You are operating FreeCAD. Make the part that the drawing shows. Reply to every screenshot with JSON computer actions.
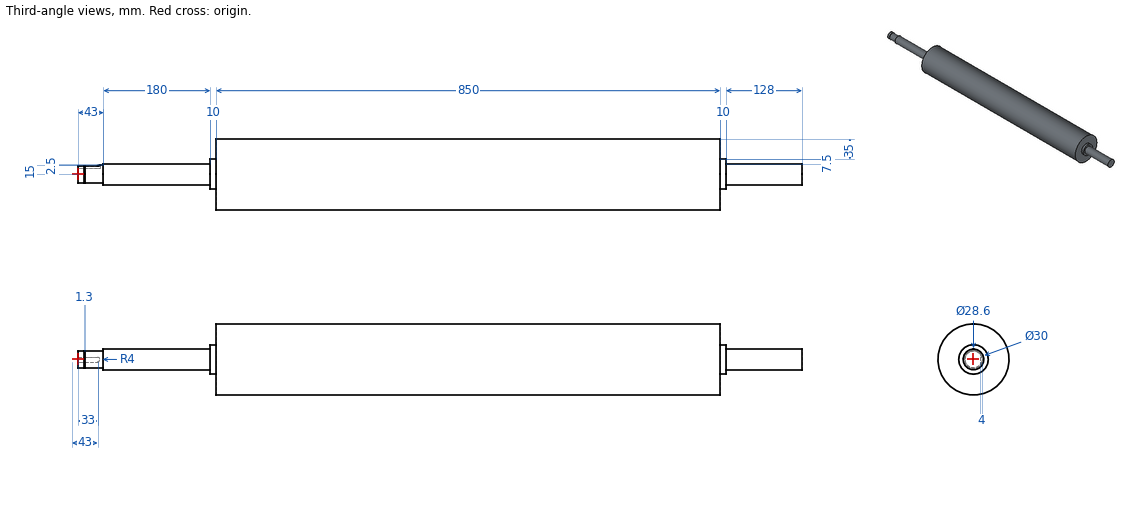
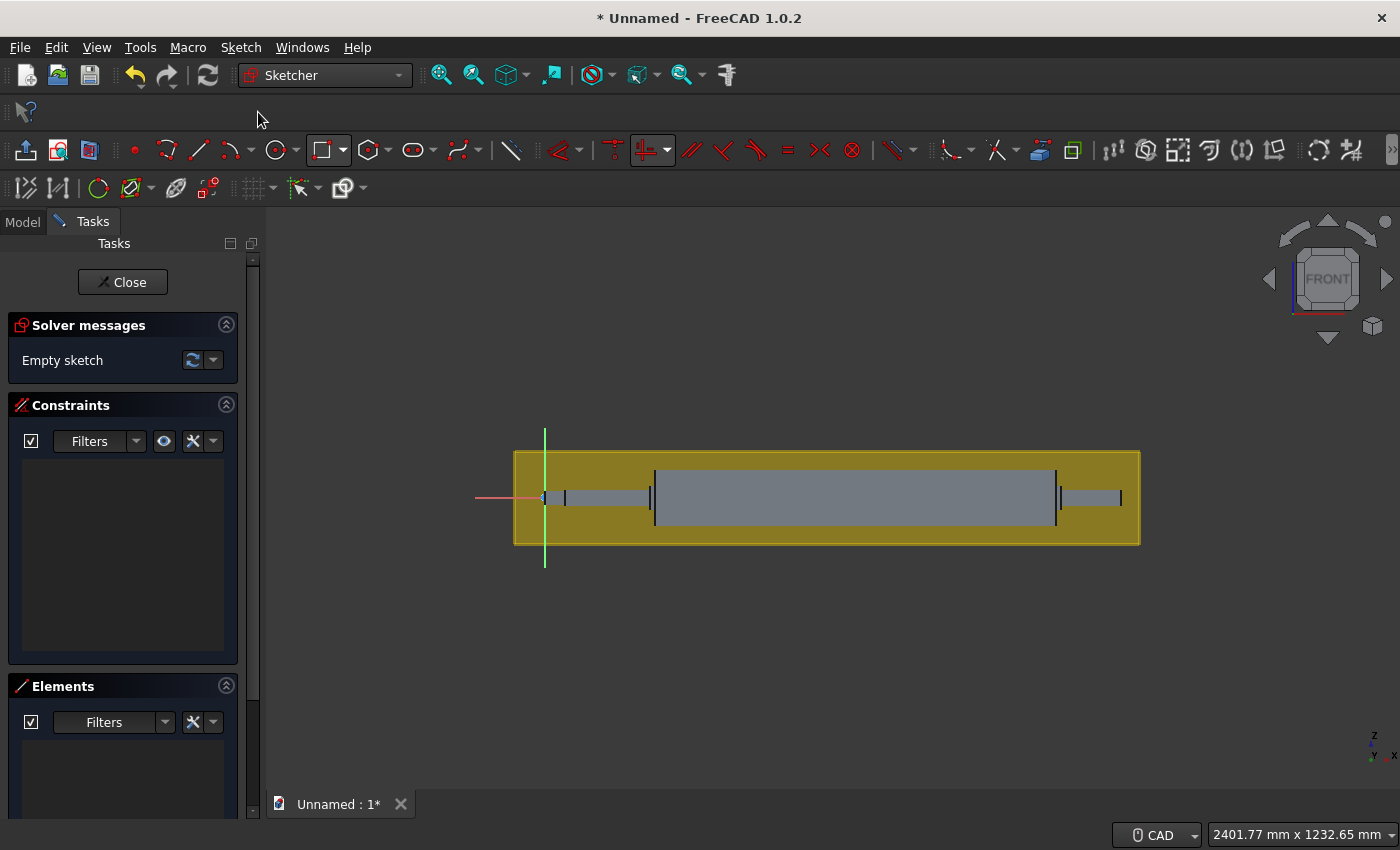
{"action": "left_click", "coordinate": [90, 150]}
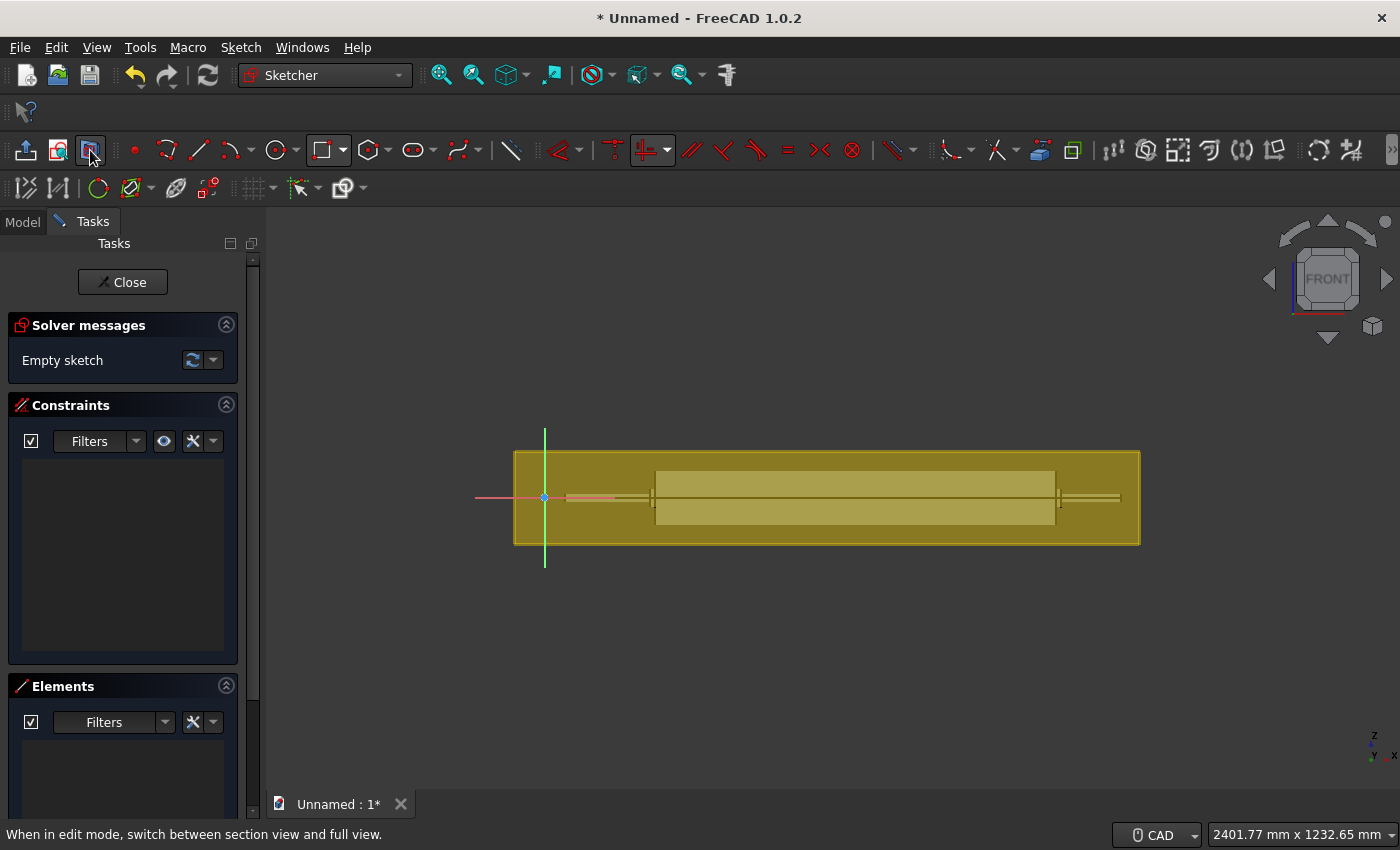
{"action": "scroll", "coordinate": [540, 498], "scroll_direction": "up", "scroll_amount": 15}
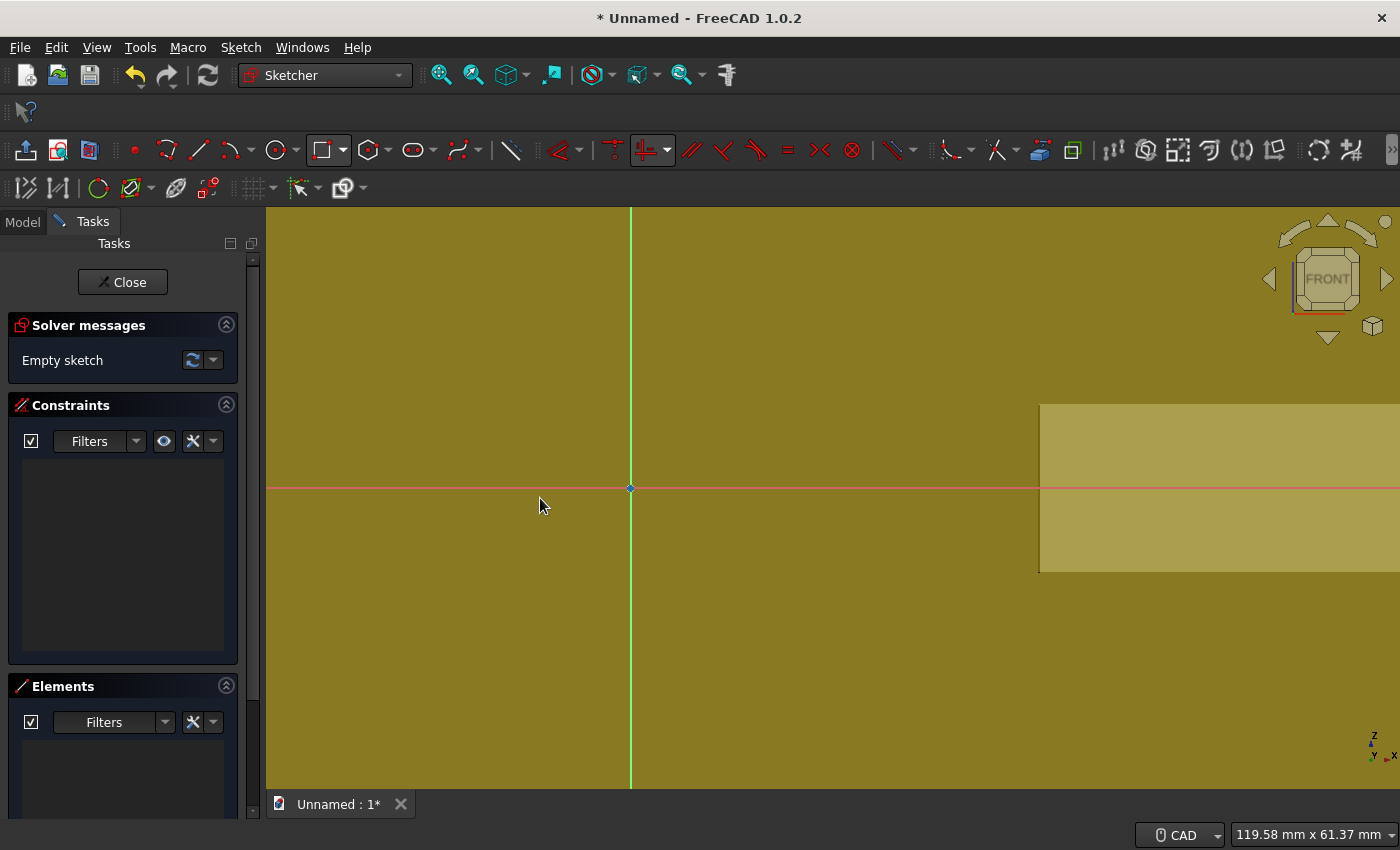
{"action": "scroll", "coordinate": [747, 469], "scroll_direction": "up", "scroll_amount": 2}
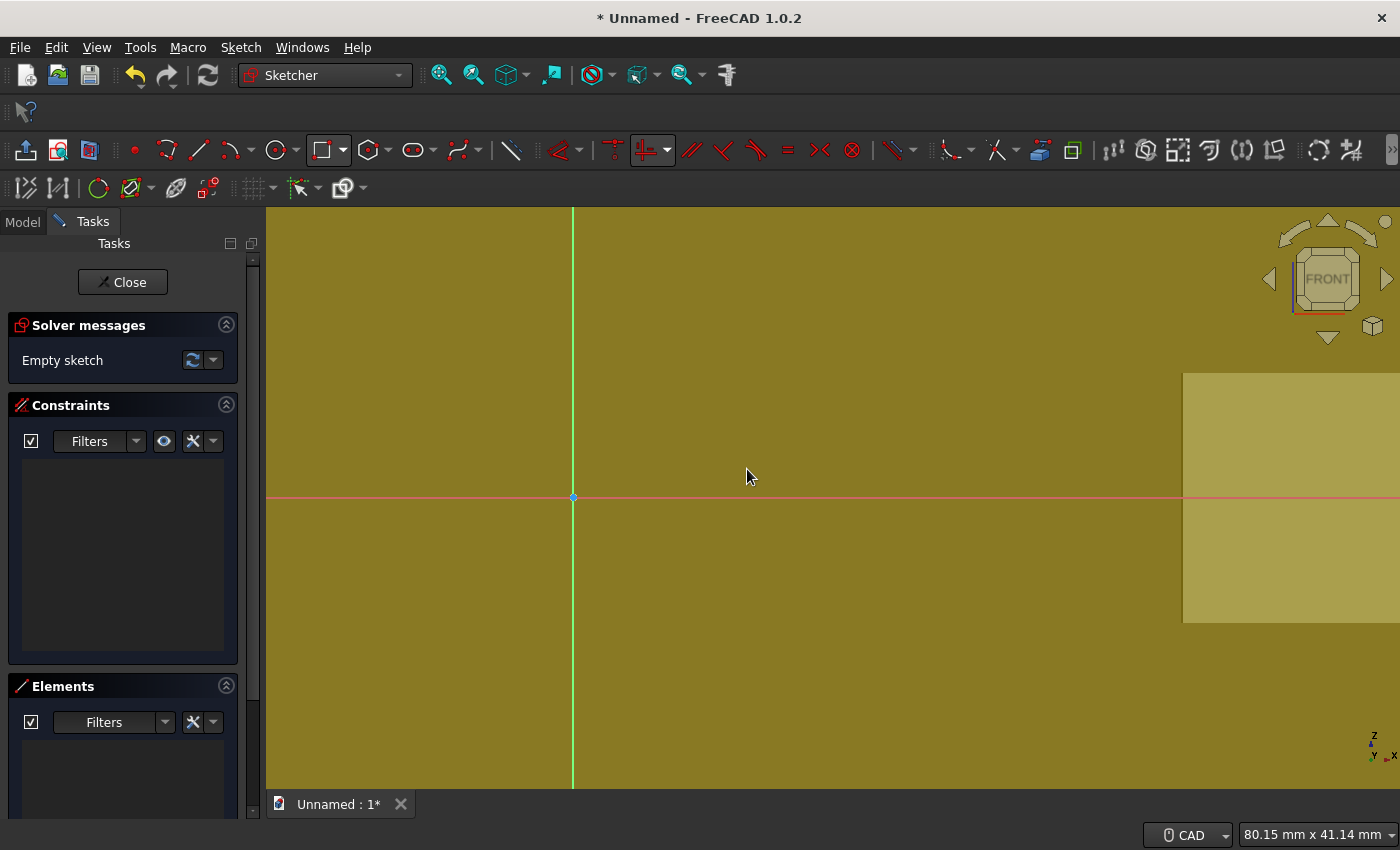
{"action": "key", "text": "g m"}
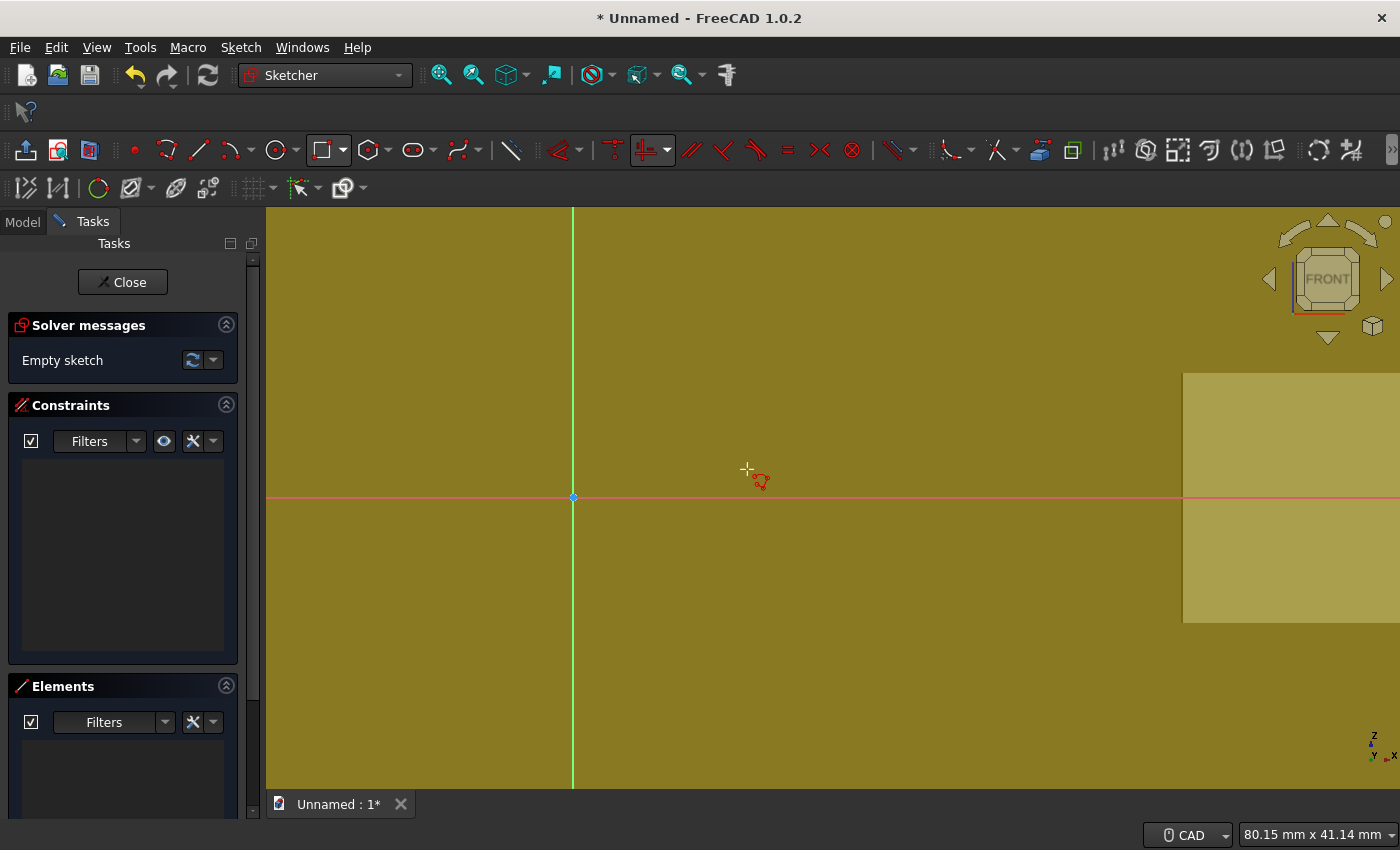
{"action": "left_click", "coordinate": [1040, 554]}
{"action": "left_click", "coordinate": [432, 554]}
{"action": "left_click", "coordinate": [432, 441]}
{"action": "left_click", "coordinate": [1040, 441]}
{"action": "right_click", "coordinate": [1040, 441]}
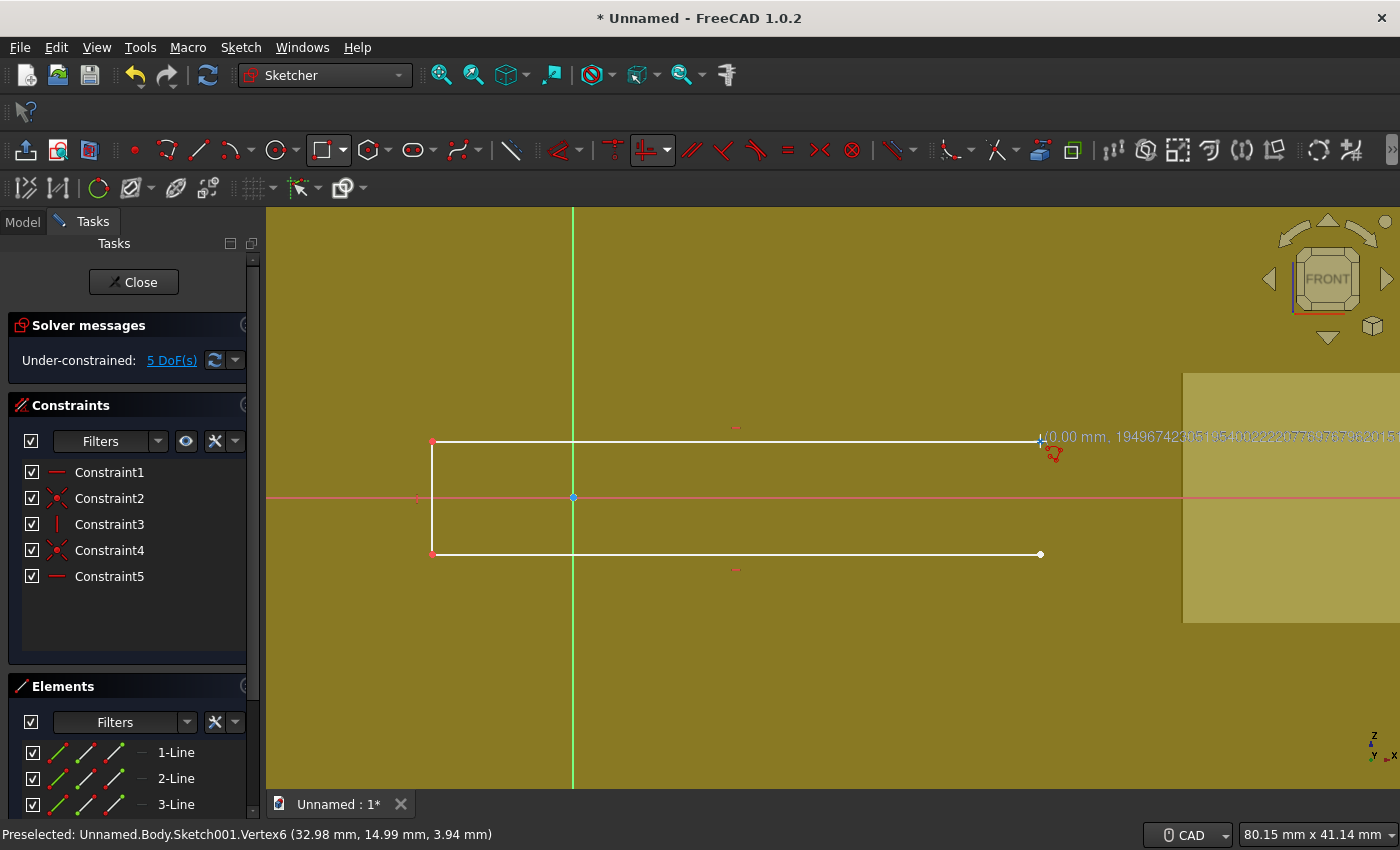
{"action": "left_click", "coordinate": [254, 150]}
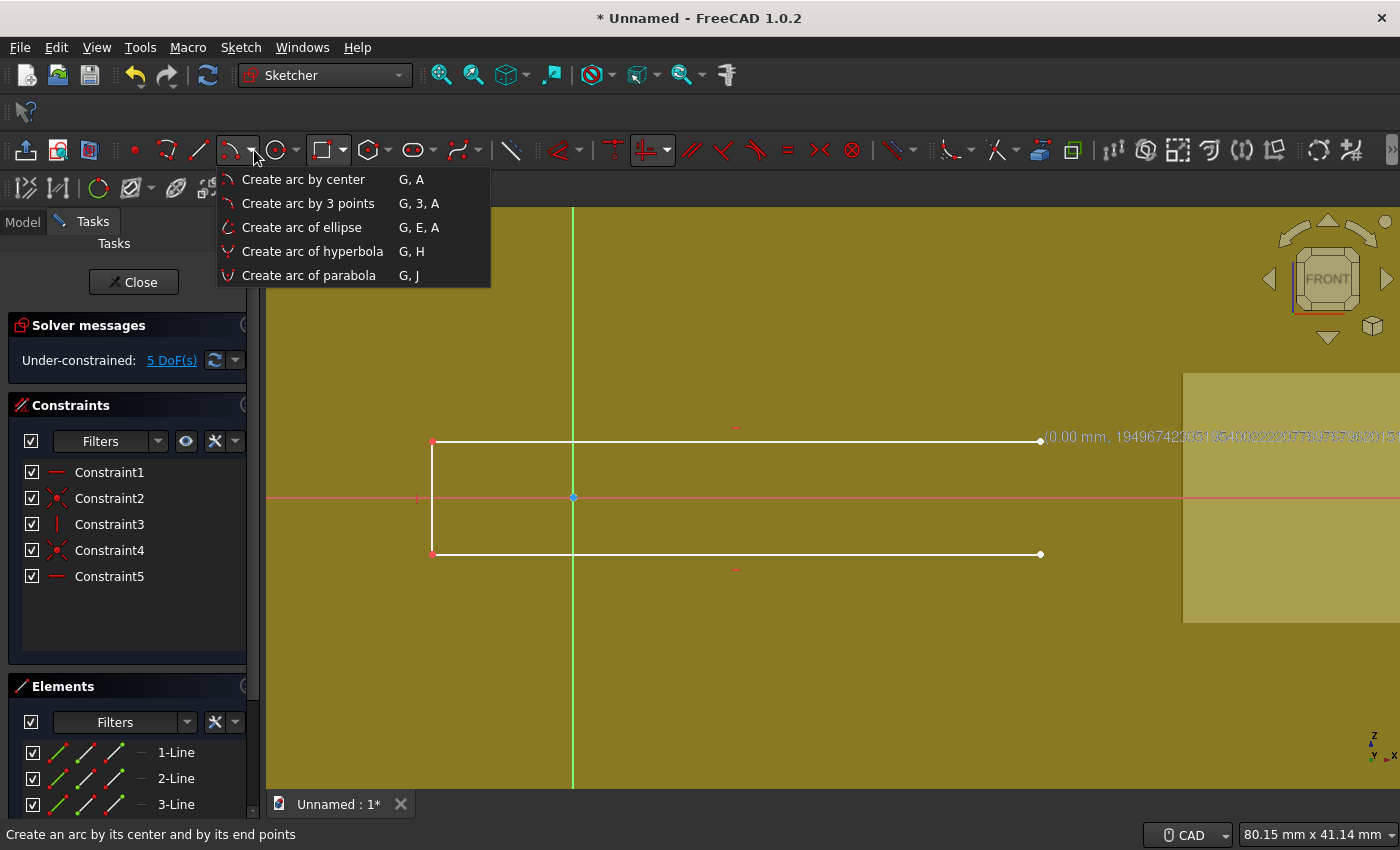
{"action": "left_click", "coordinate": [354, 203]}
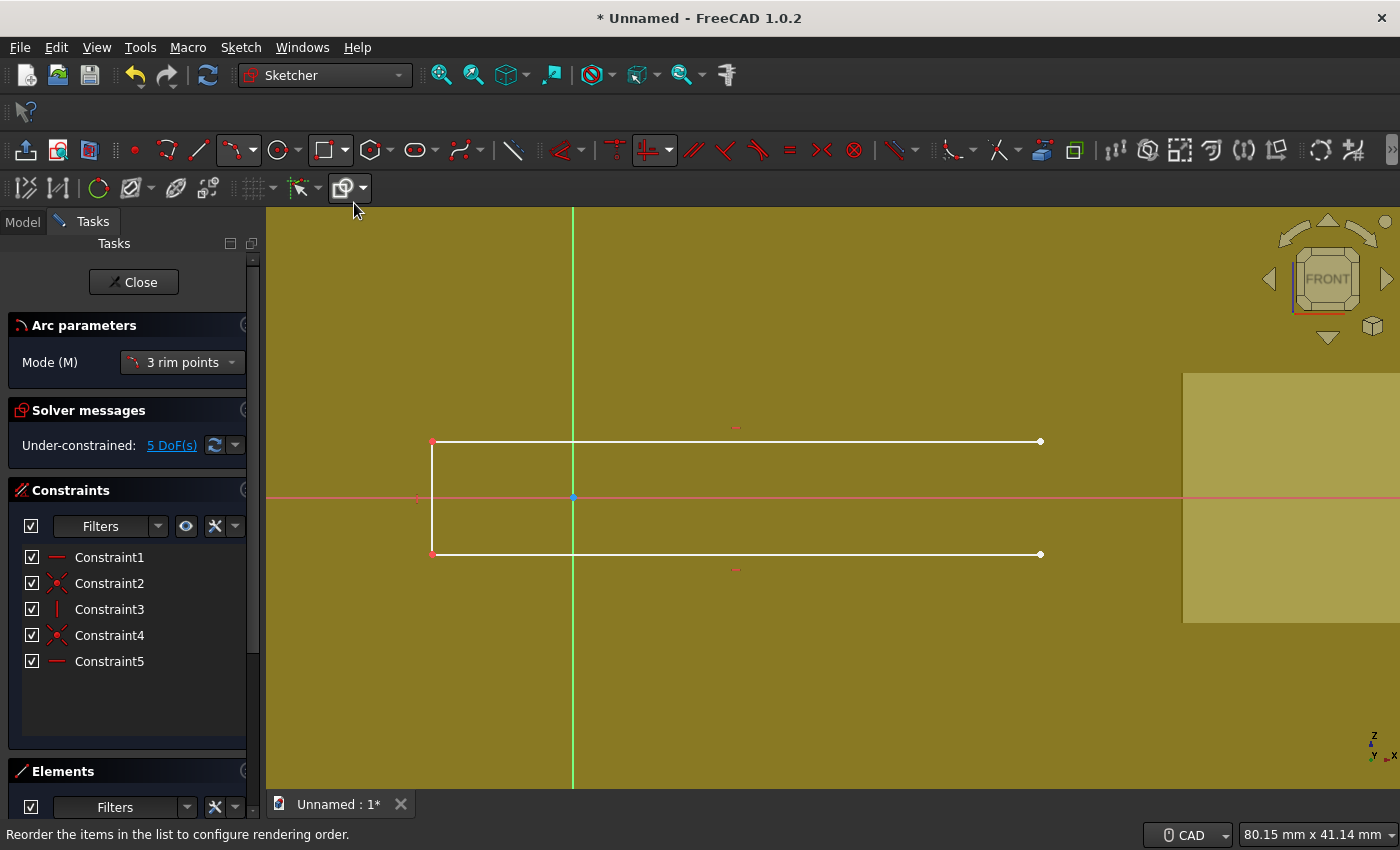
{"action": "left_click", "coordinate": [1040, 442]}
{"action": "left_click", "coordinate": [1040, 555]}
{"action": "left_click", "coordinate": [1094, 515]}
{"action": "key", "text": "Escape"}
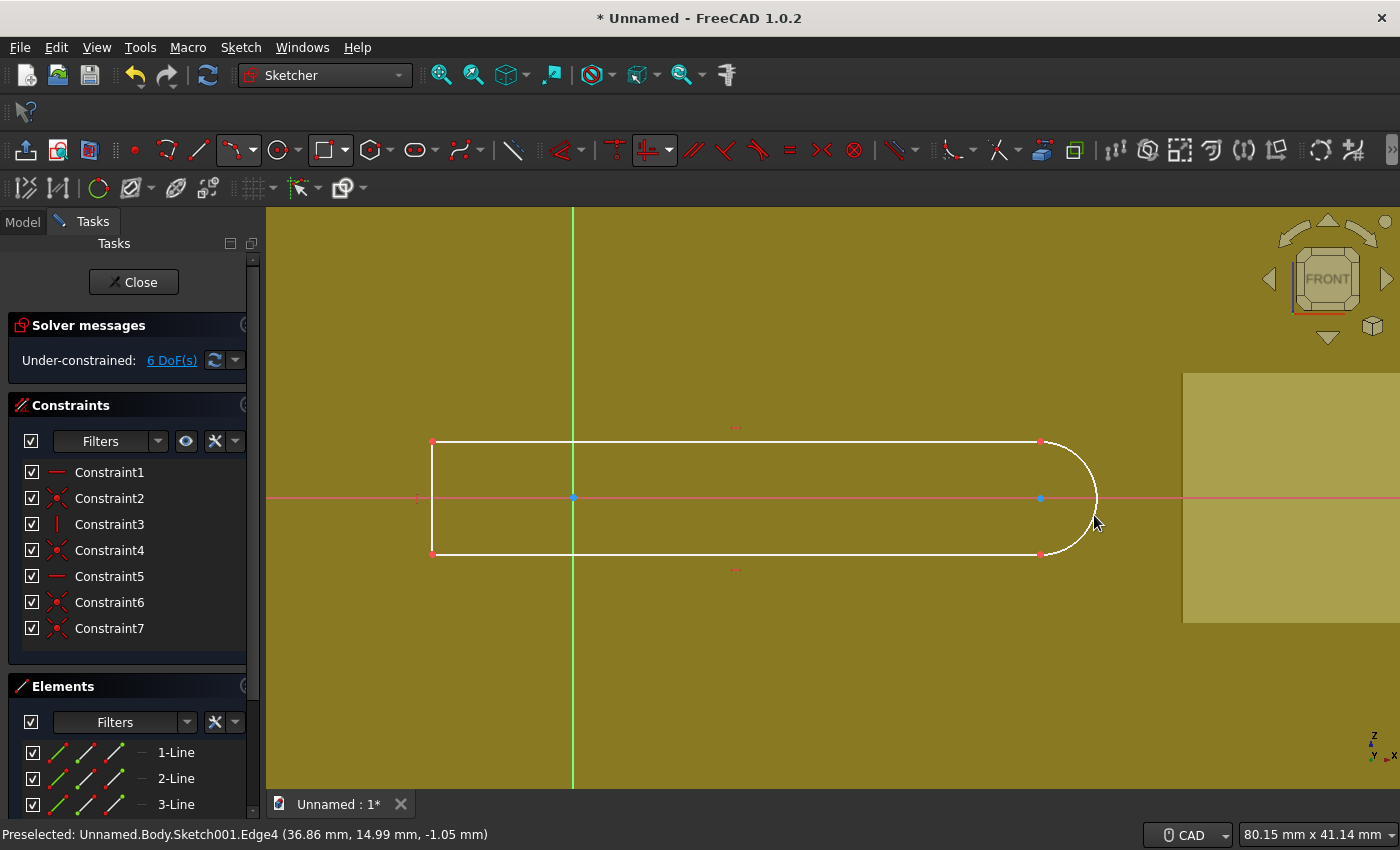
{"action": "left_click", "coordinate": [858, 555]}